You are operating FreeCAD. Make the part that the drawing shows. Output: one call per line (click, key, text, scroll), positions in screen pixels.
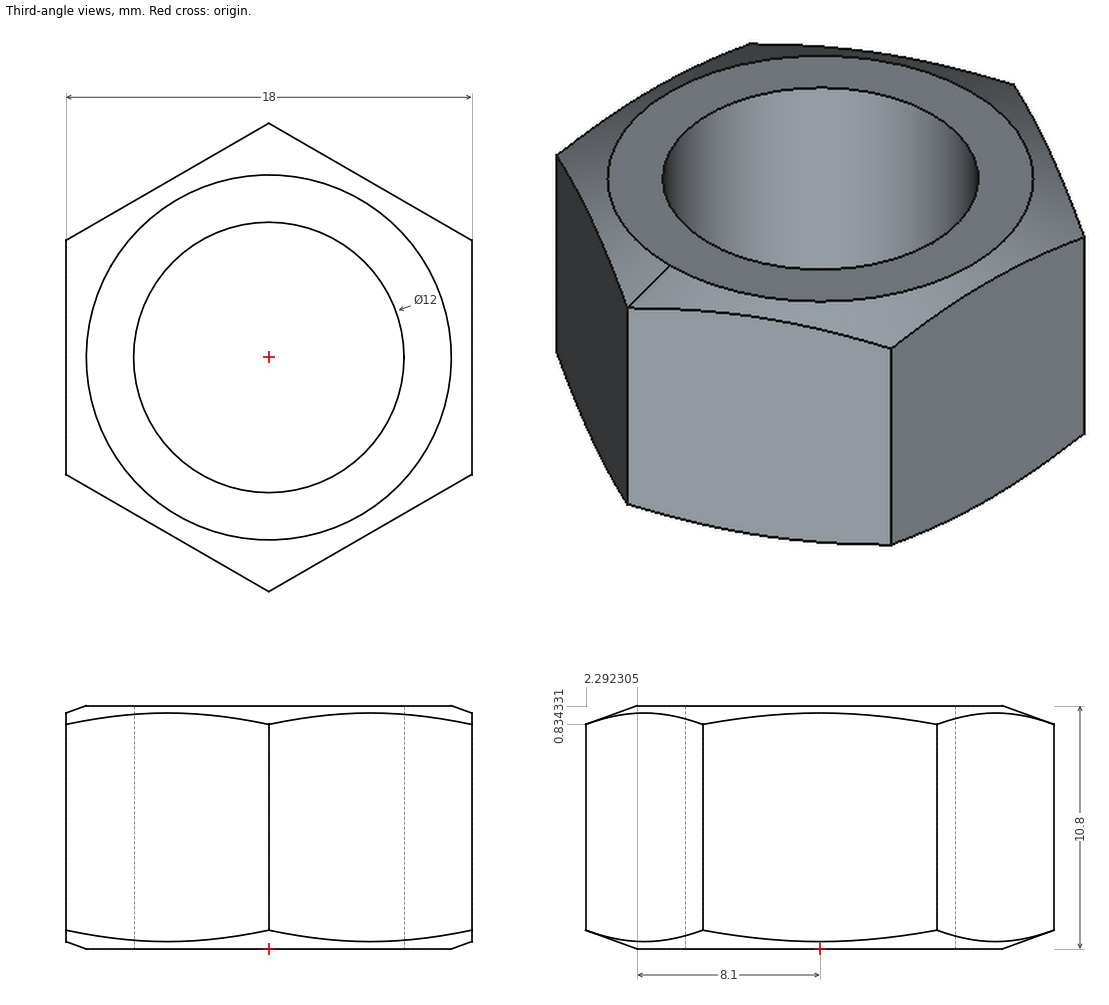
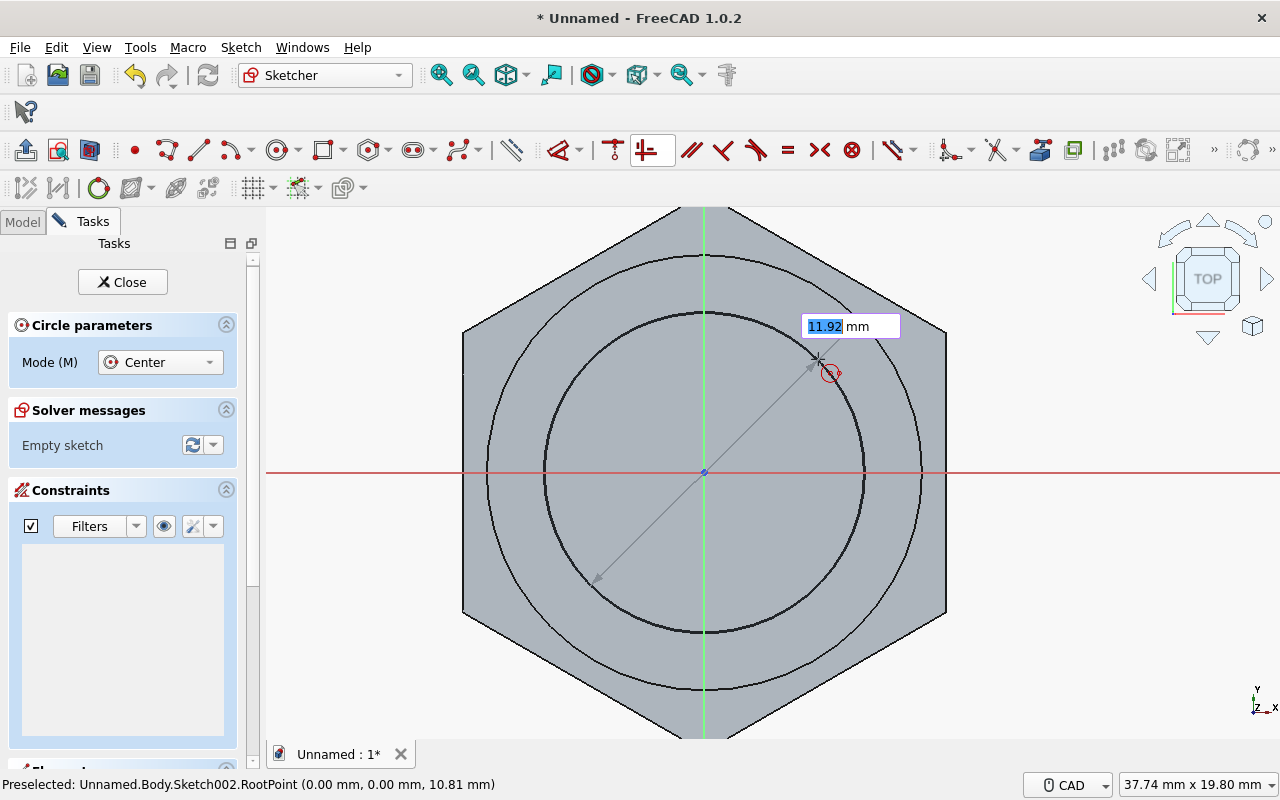
text(12)
key(Return)
key(Escape)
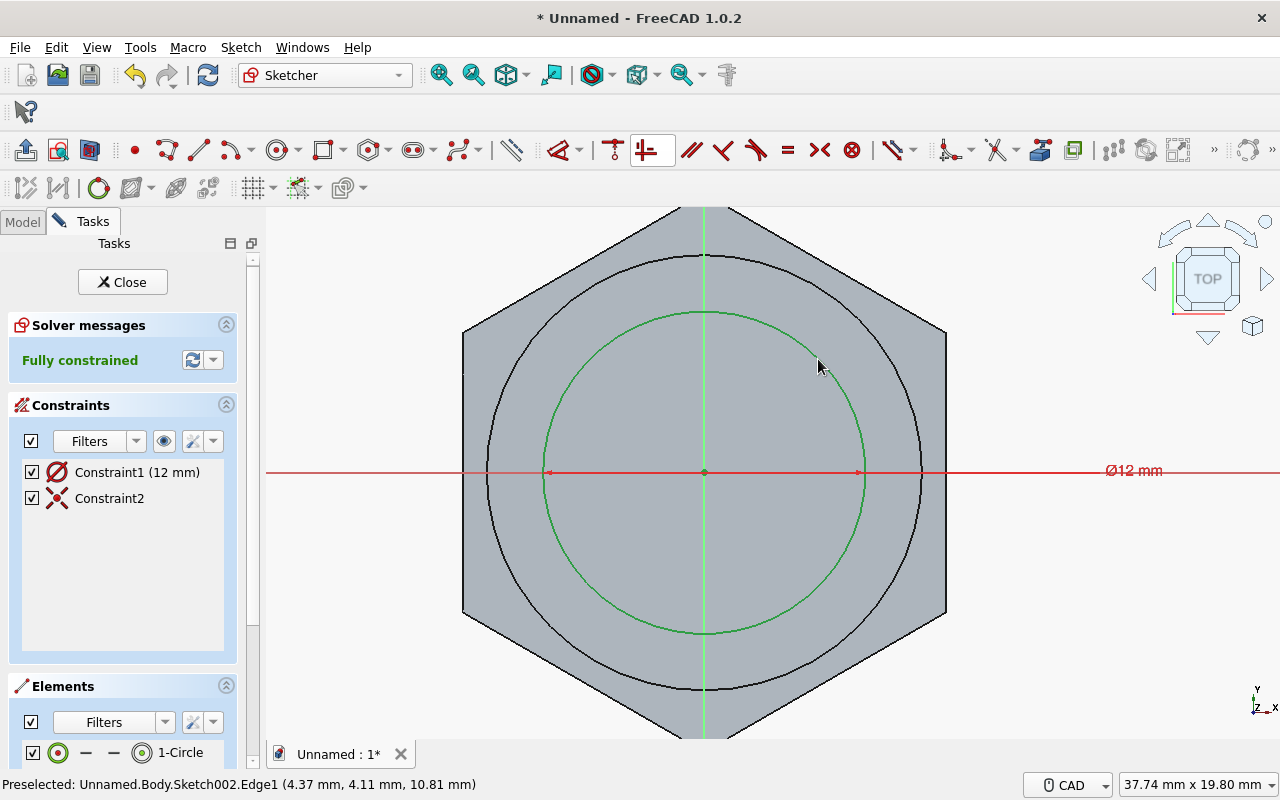
click(123, 282)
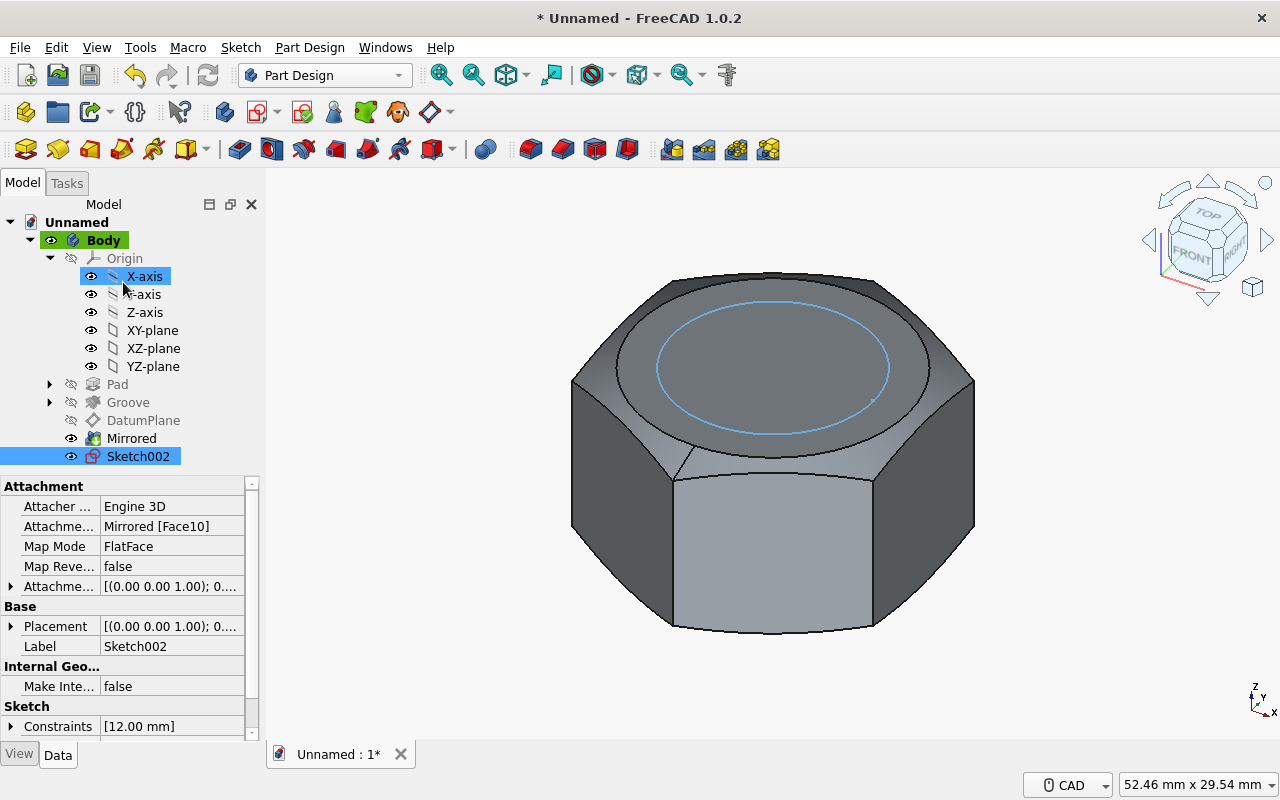
click(240, 150)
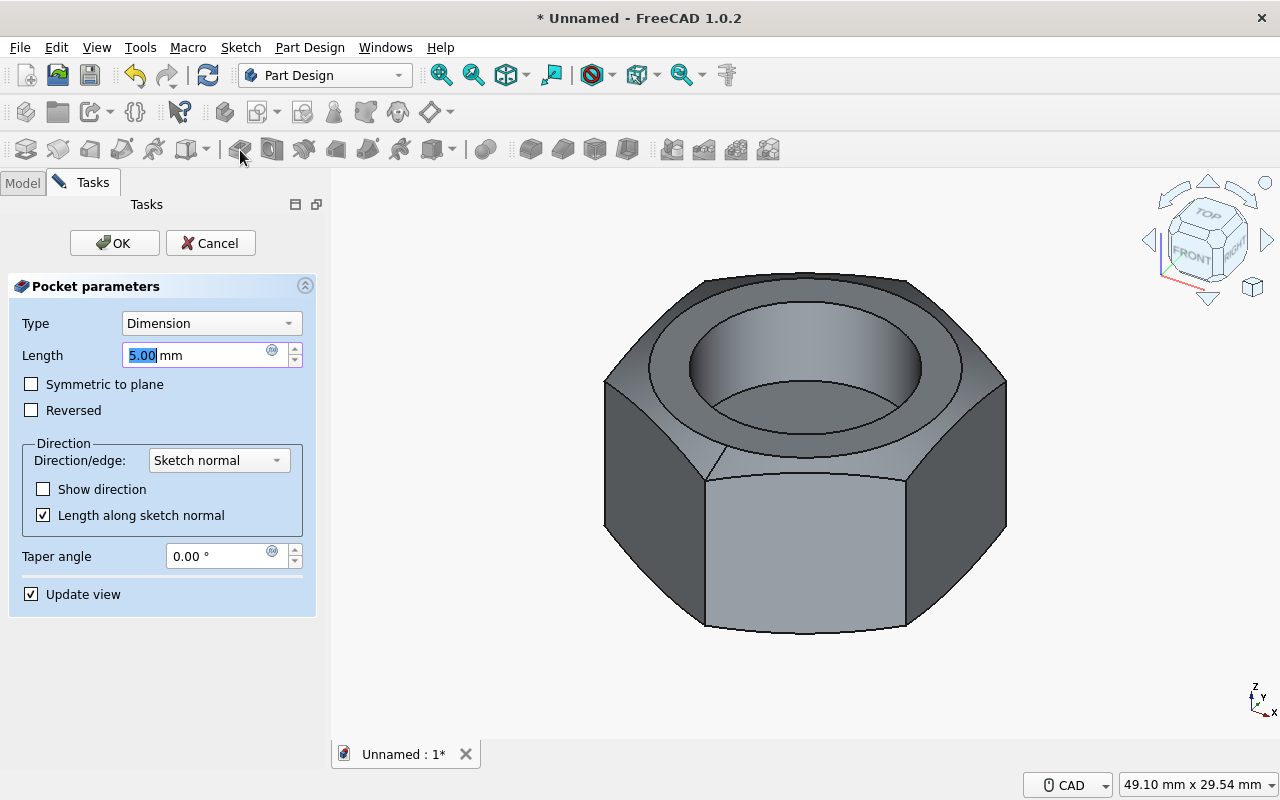
click(212, 324)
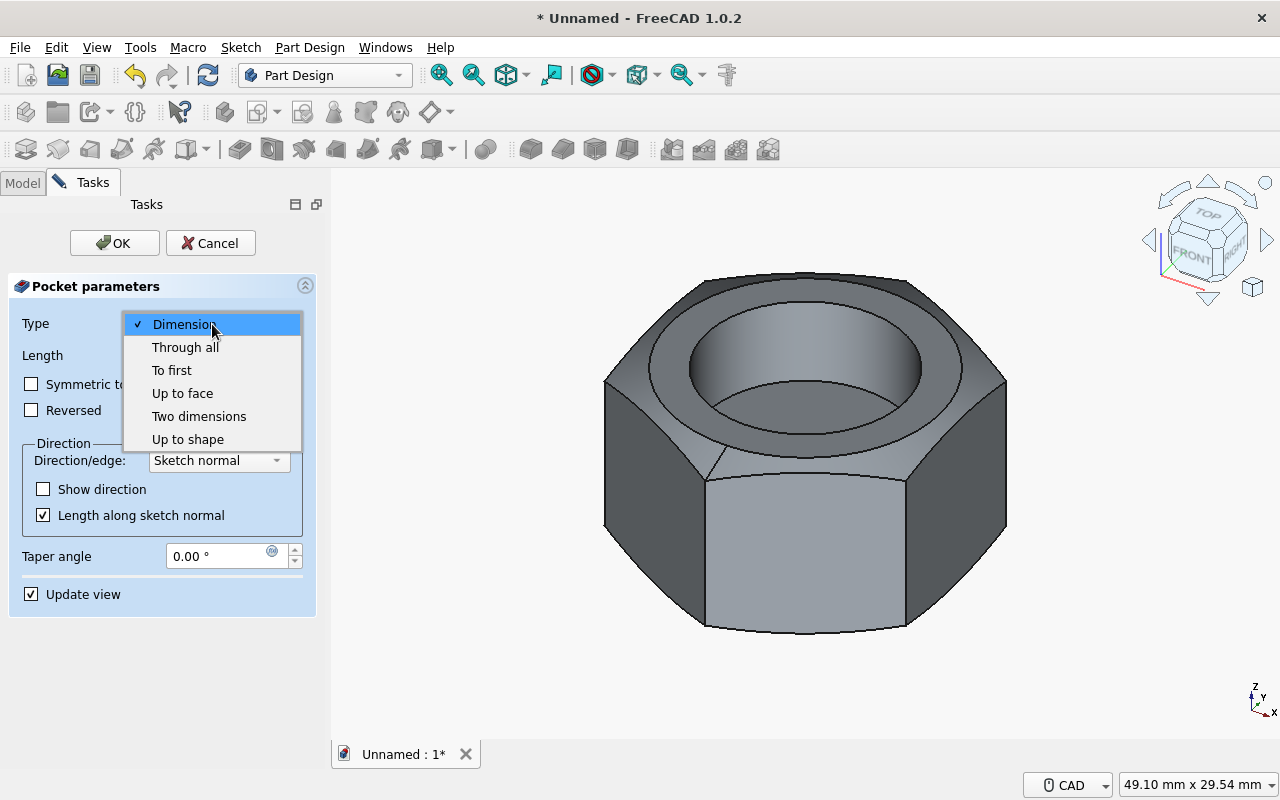
click(212, 348)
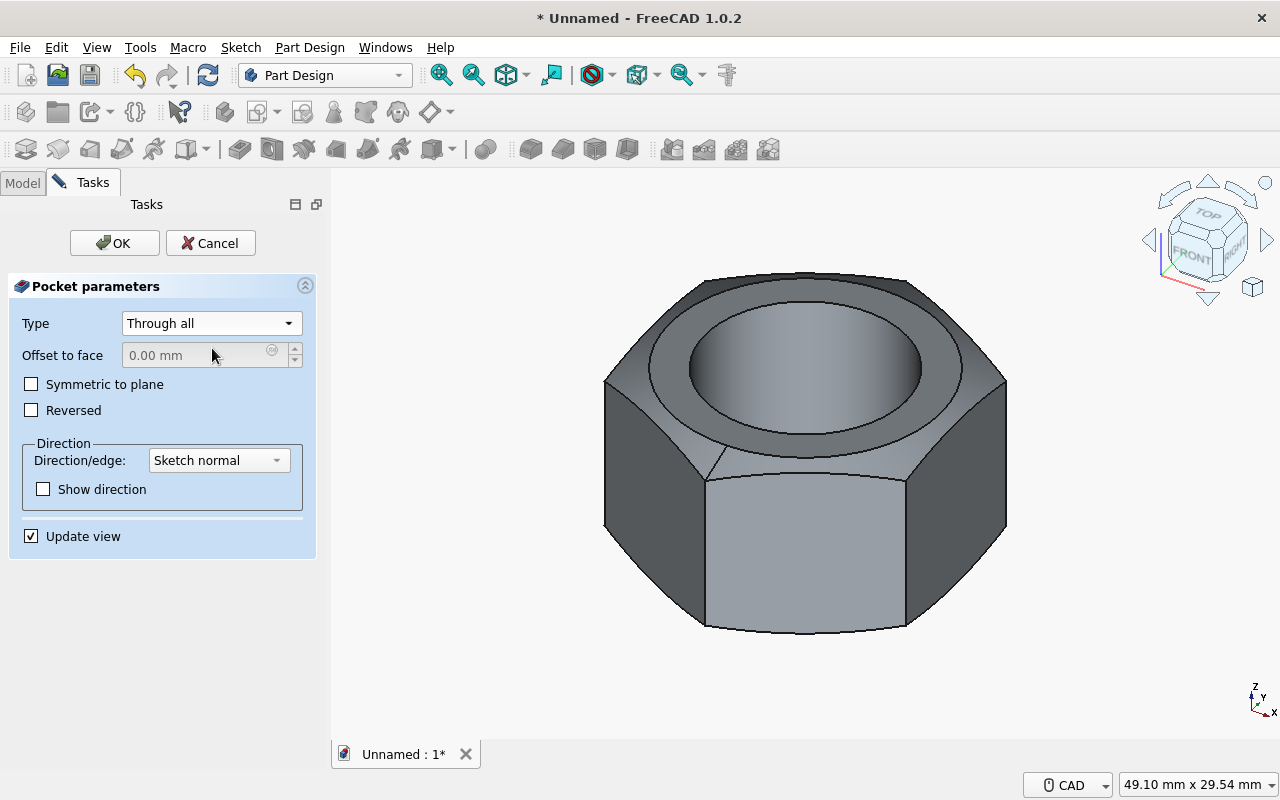
click(115, 243)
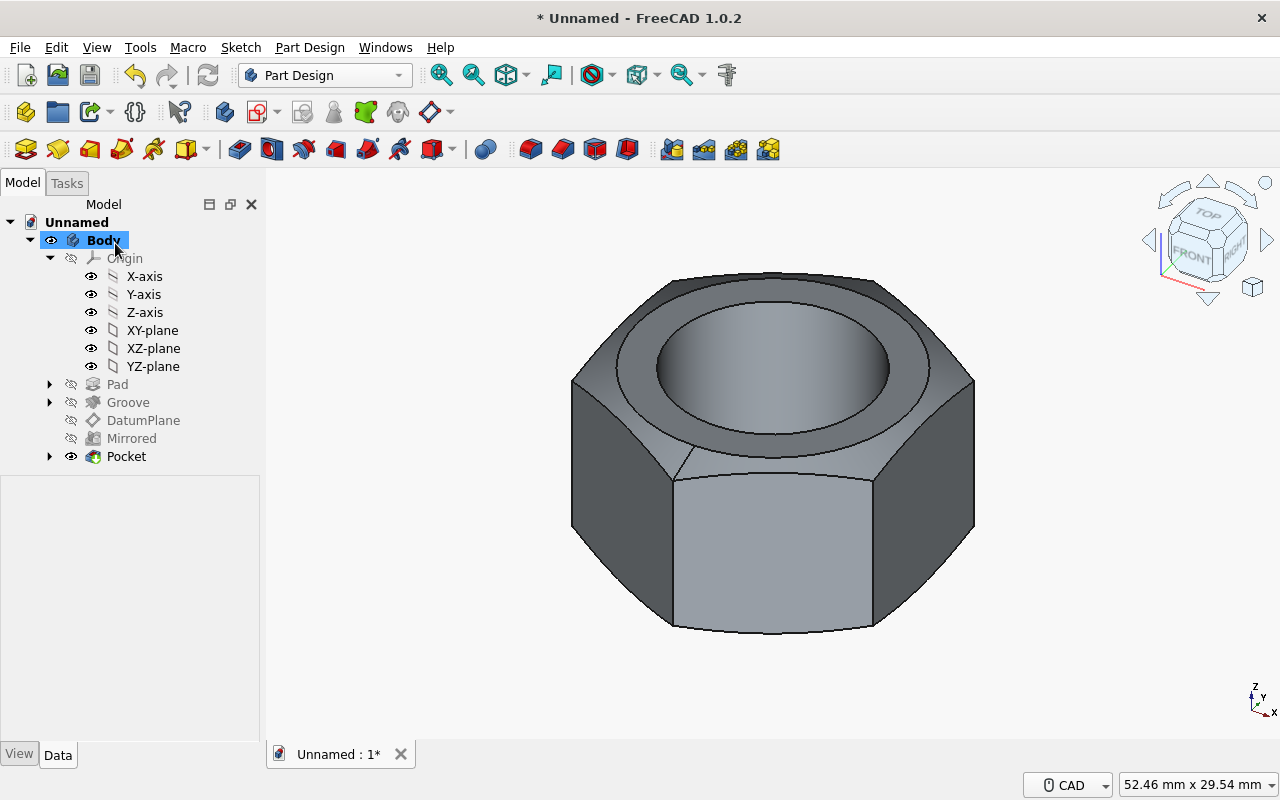
key(0)